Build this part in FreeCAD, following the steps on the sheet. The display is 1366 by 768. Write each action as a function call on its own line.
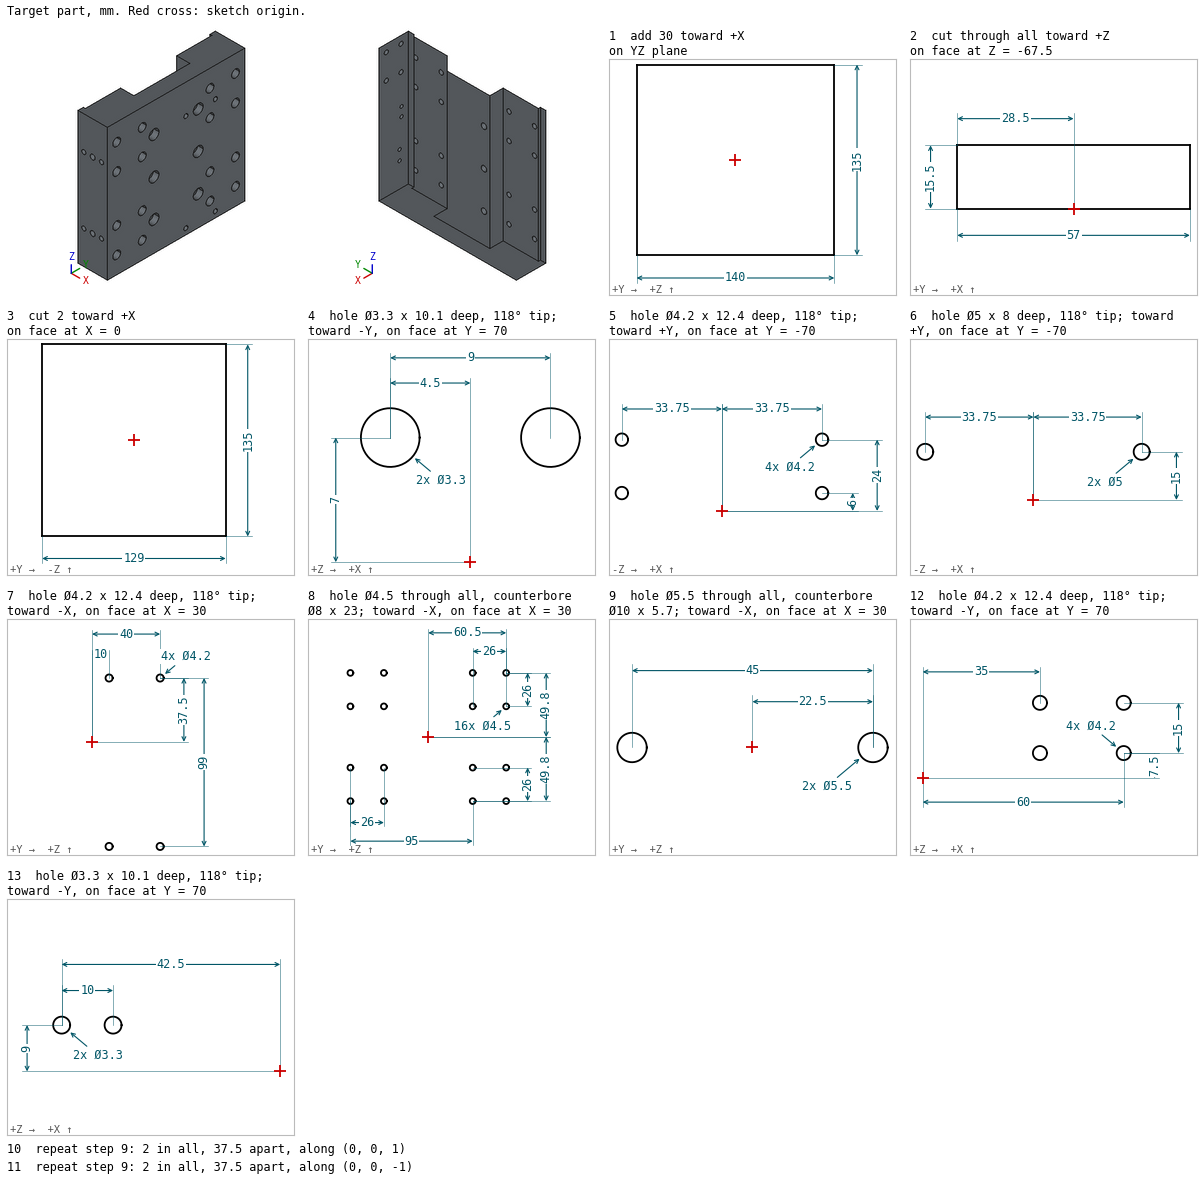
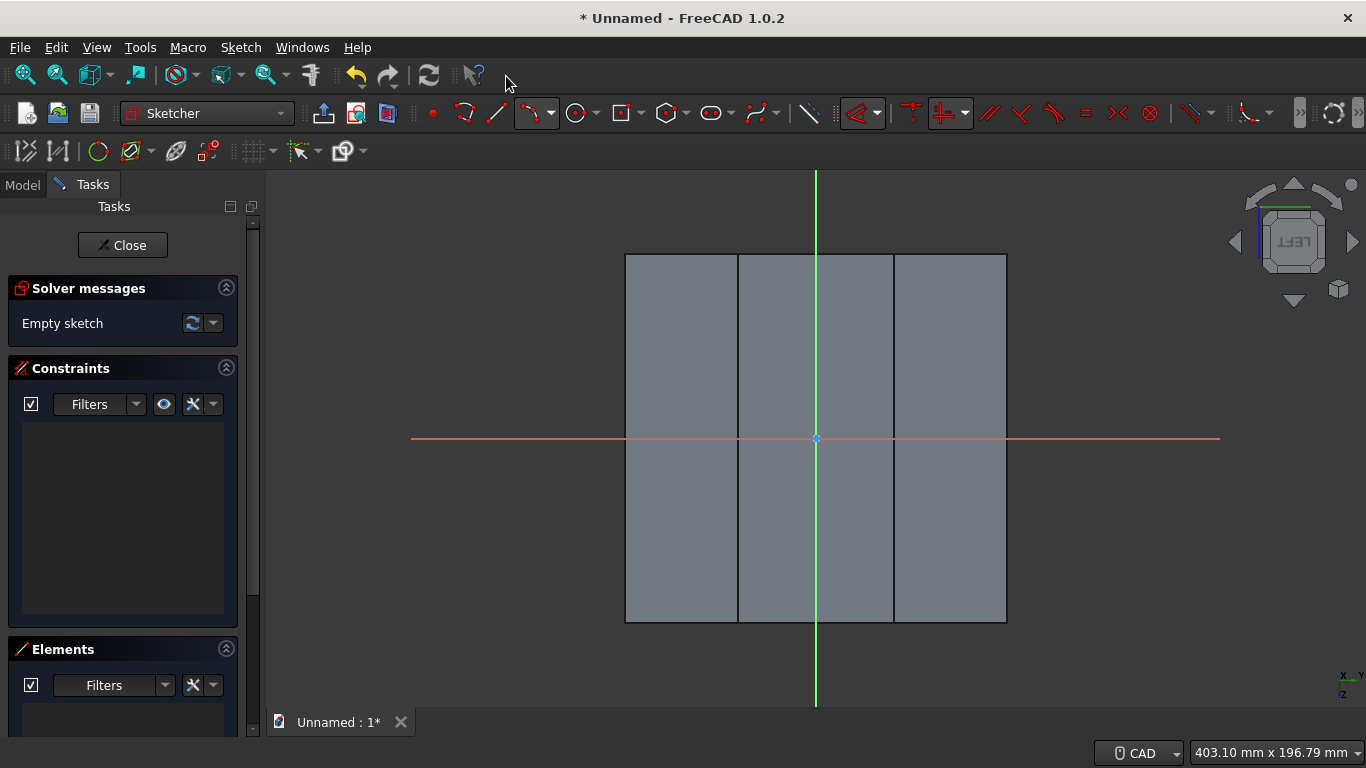
click(622, 114)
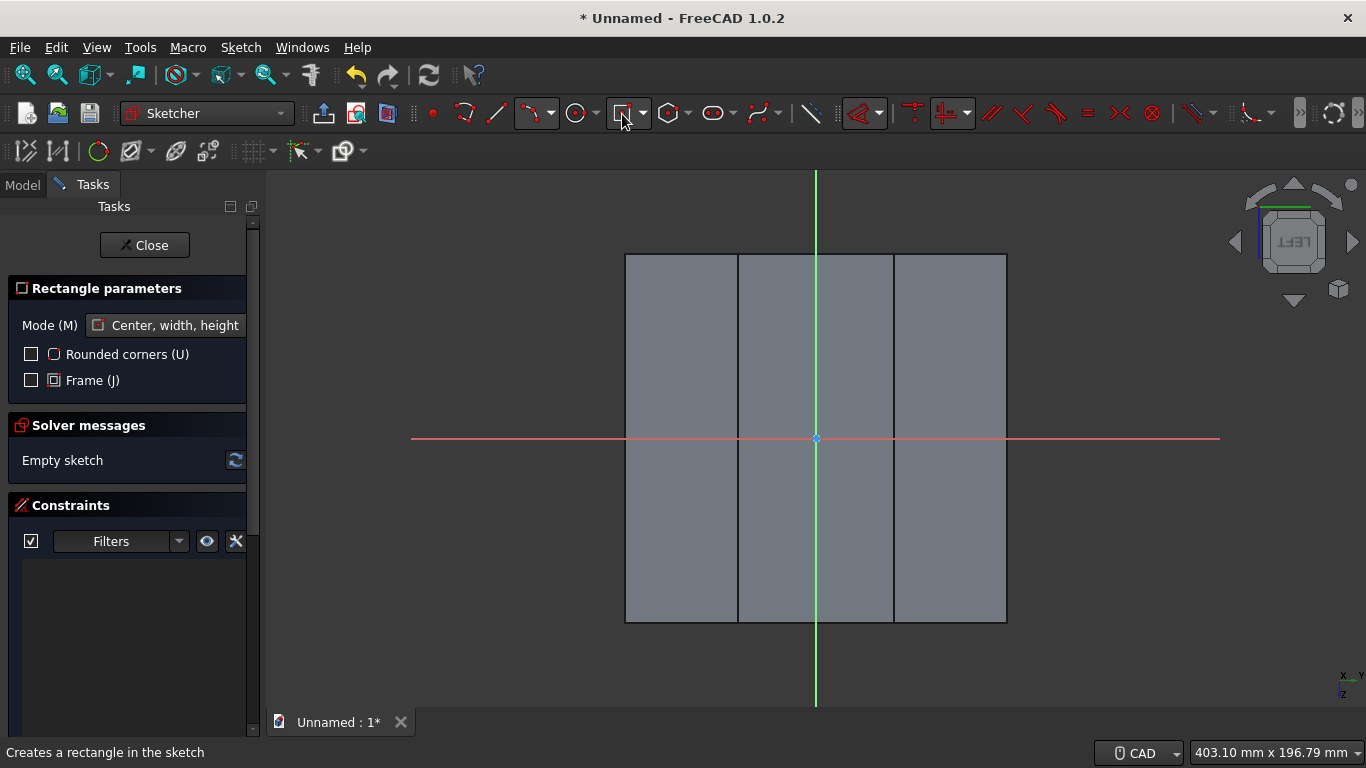
click(816, 438)
click(992, 254)
key(Escape)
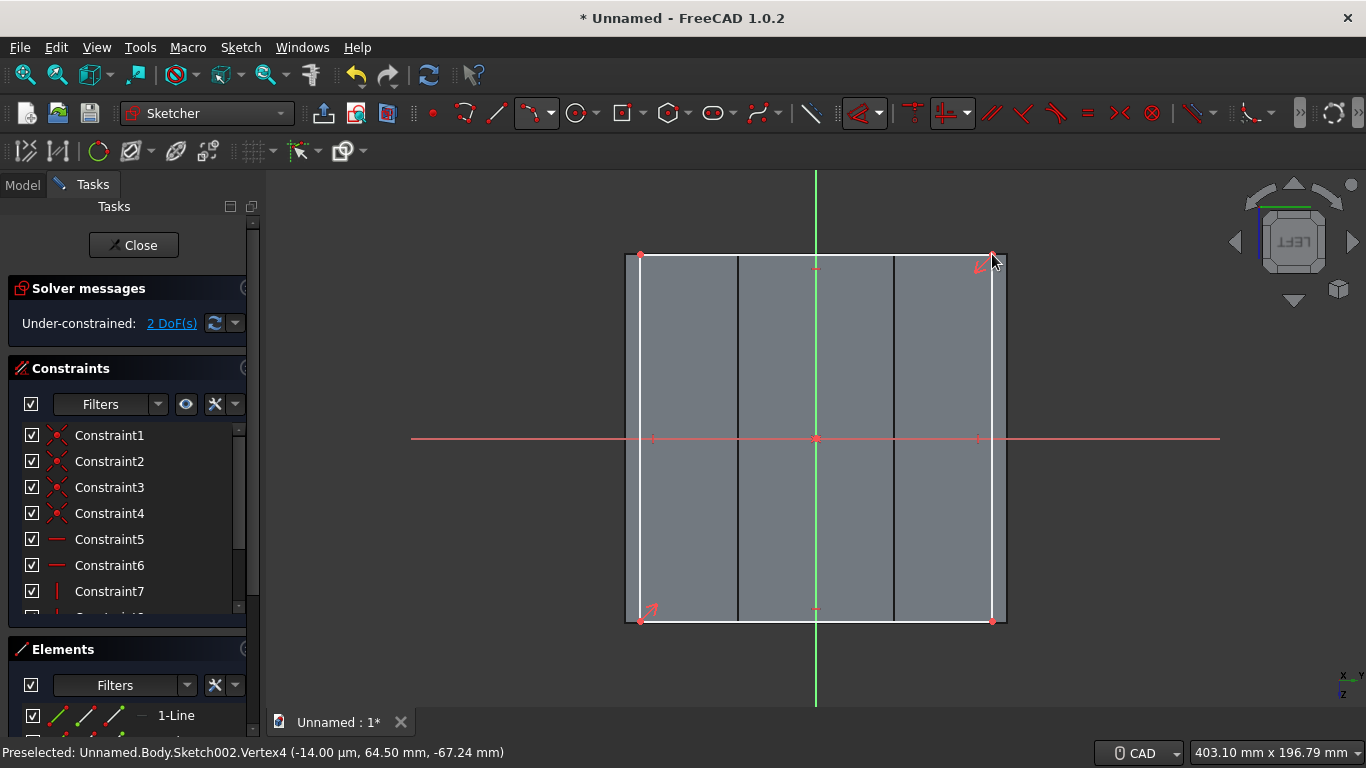
click(746, 622)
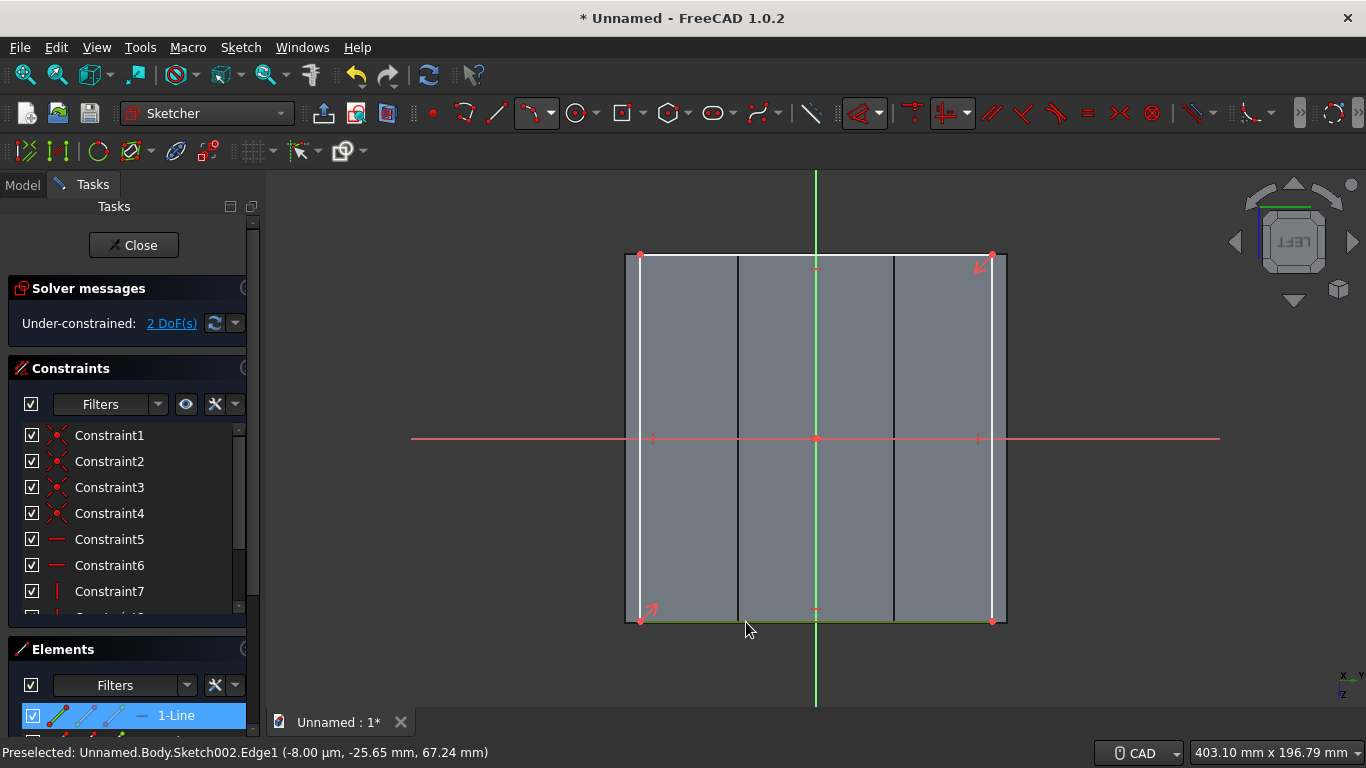
click(882, 114)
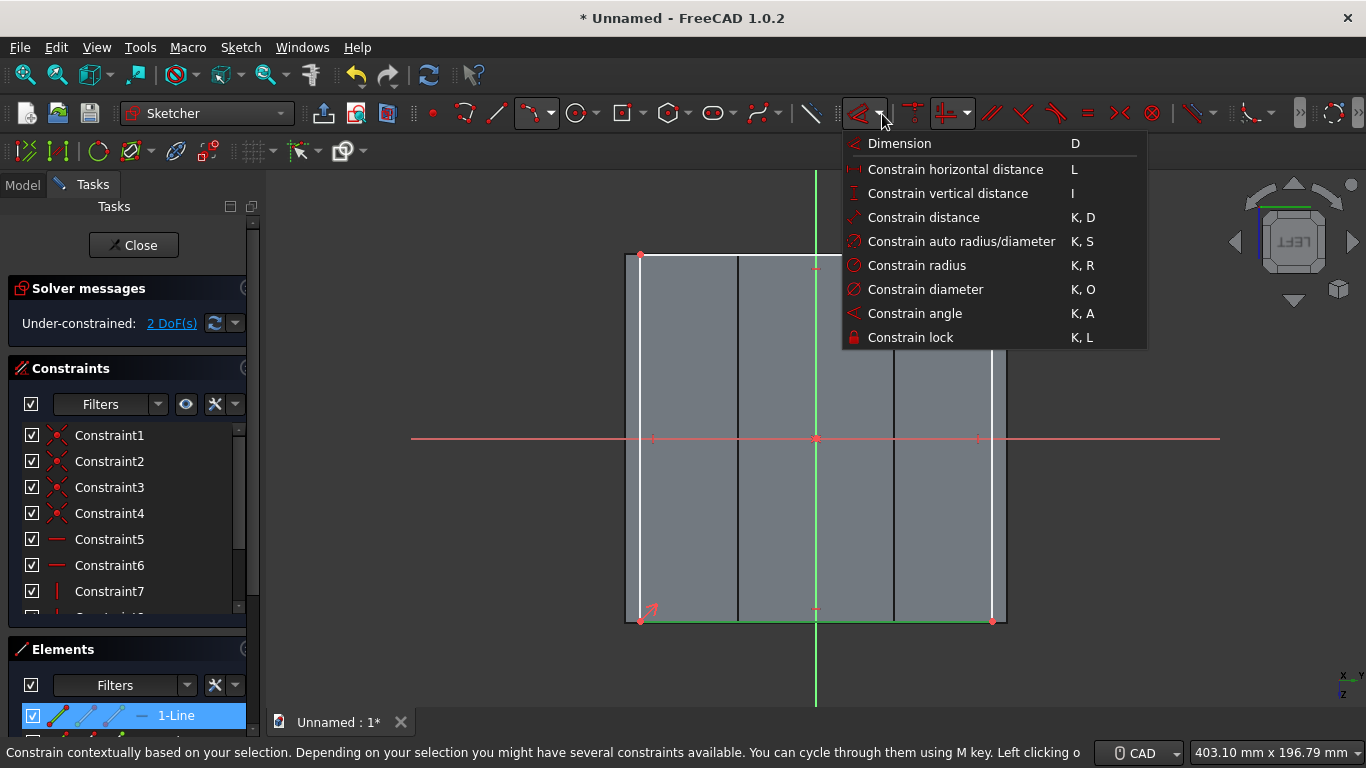
click(995, 169)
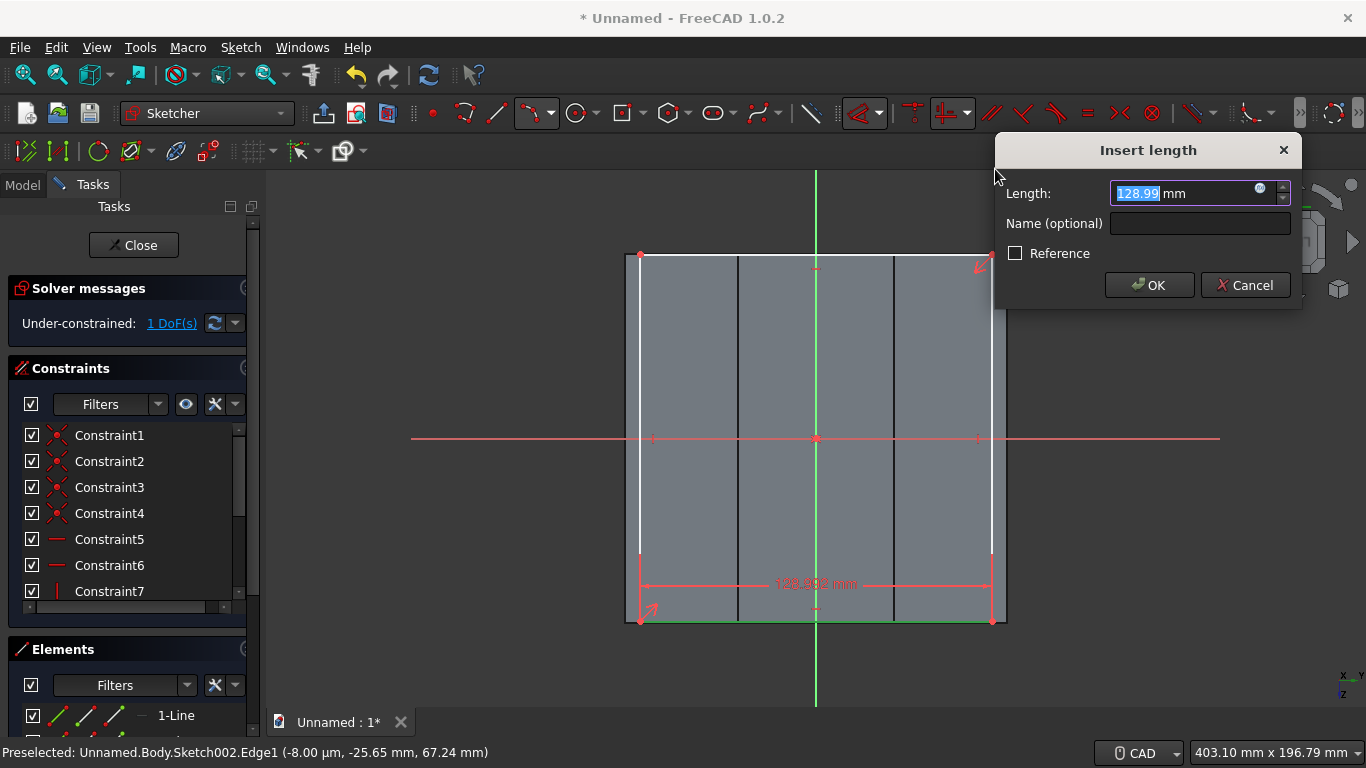
text(129)
key(Return)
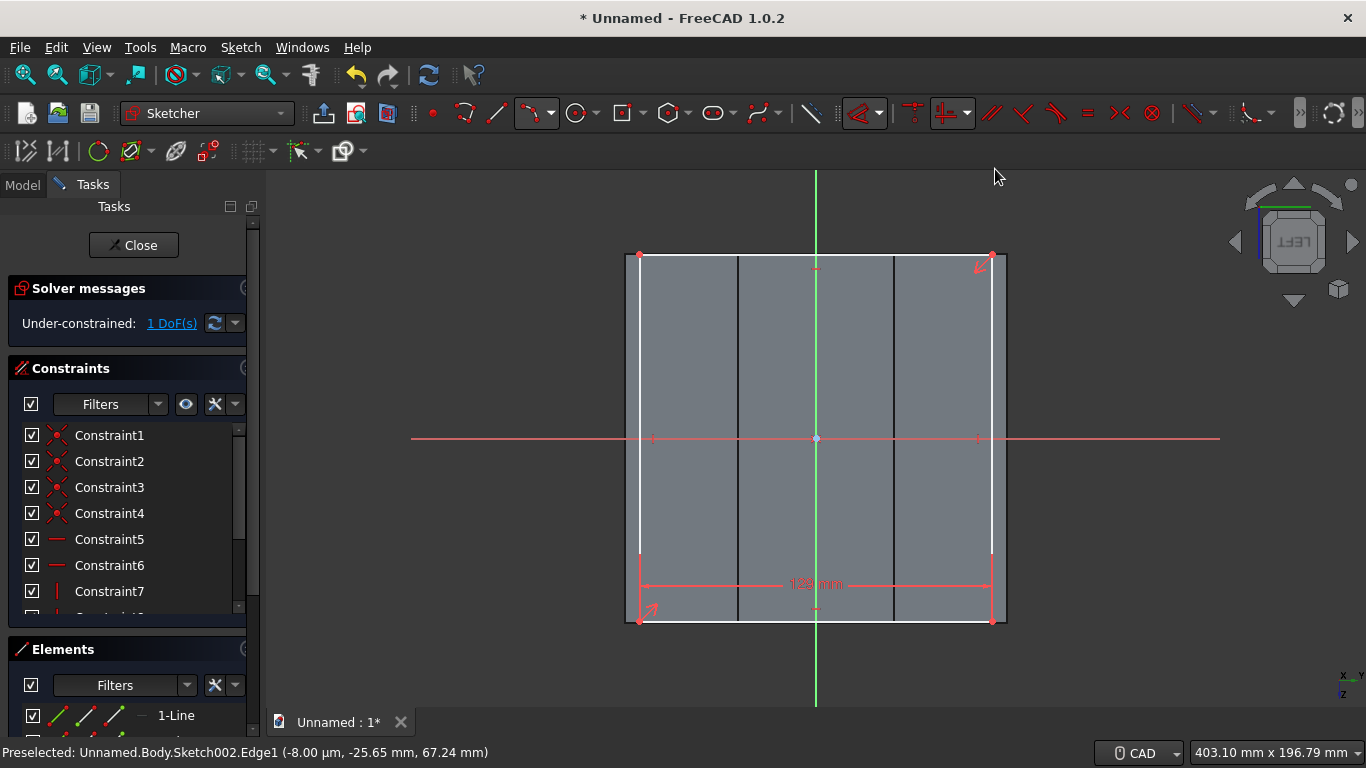
click(992, 512)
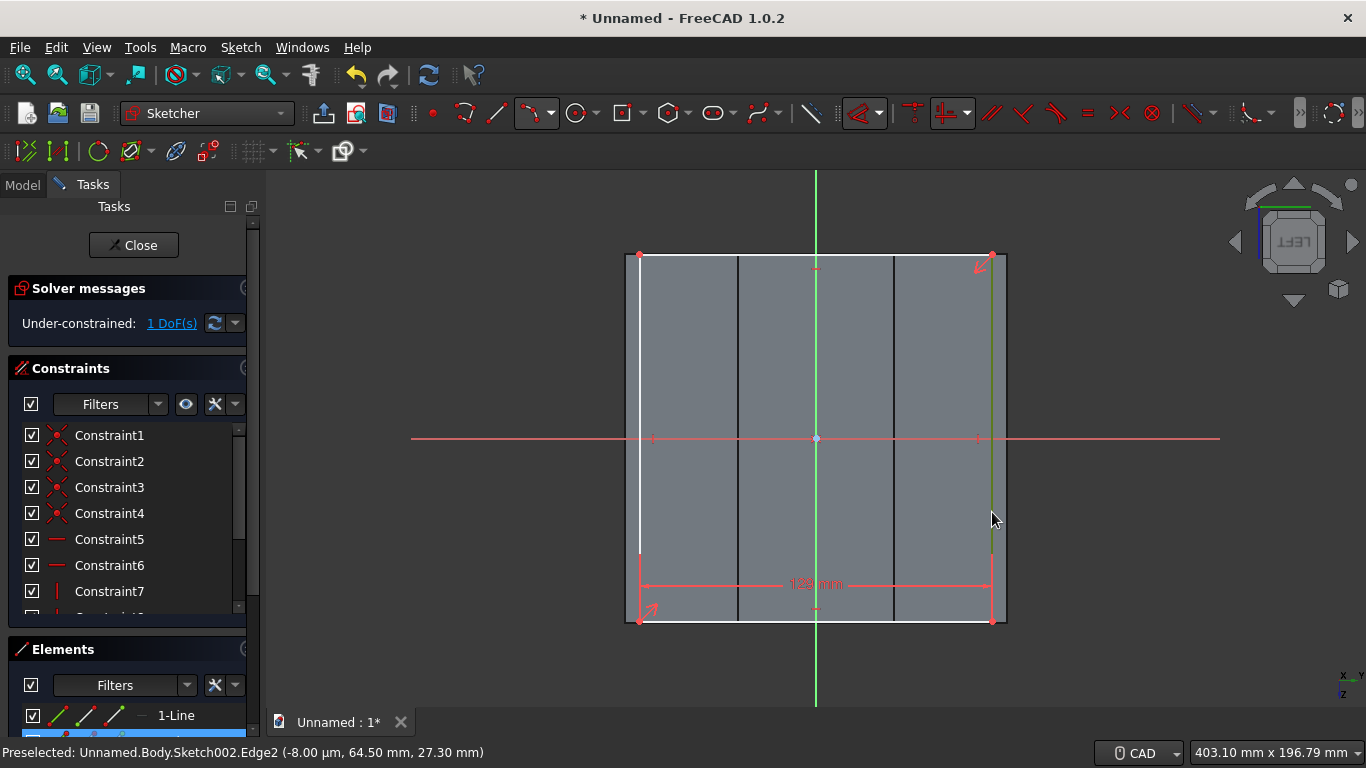
click(882, 114)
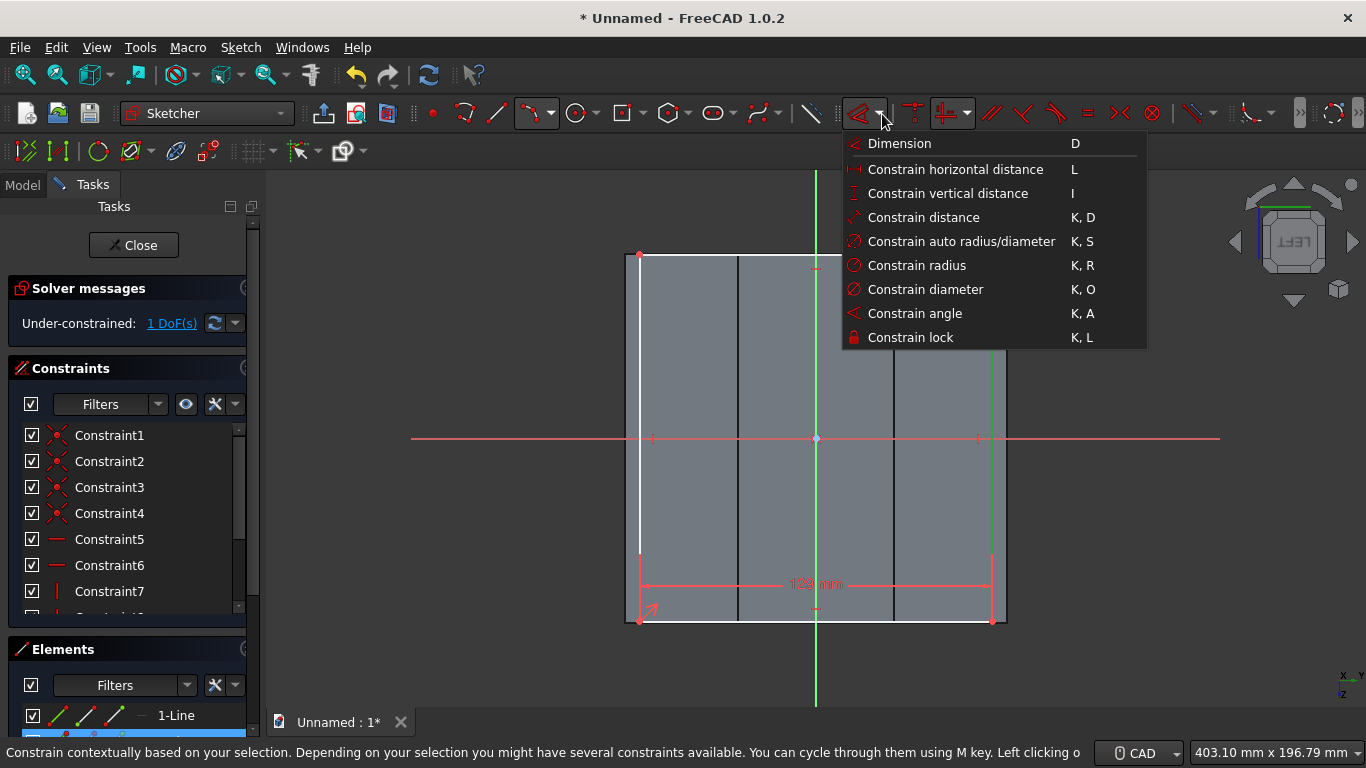
click(995, 193)